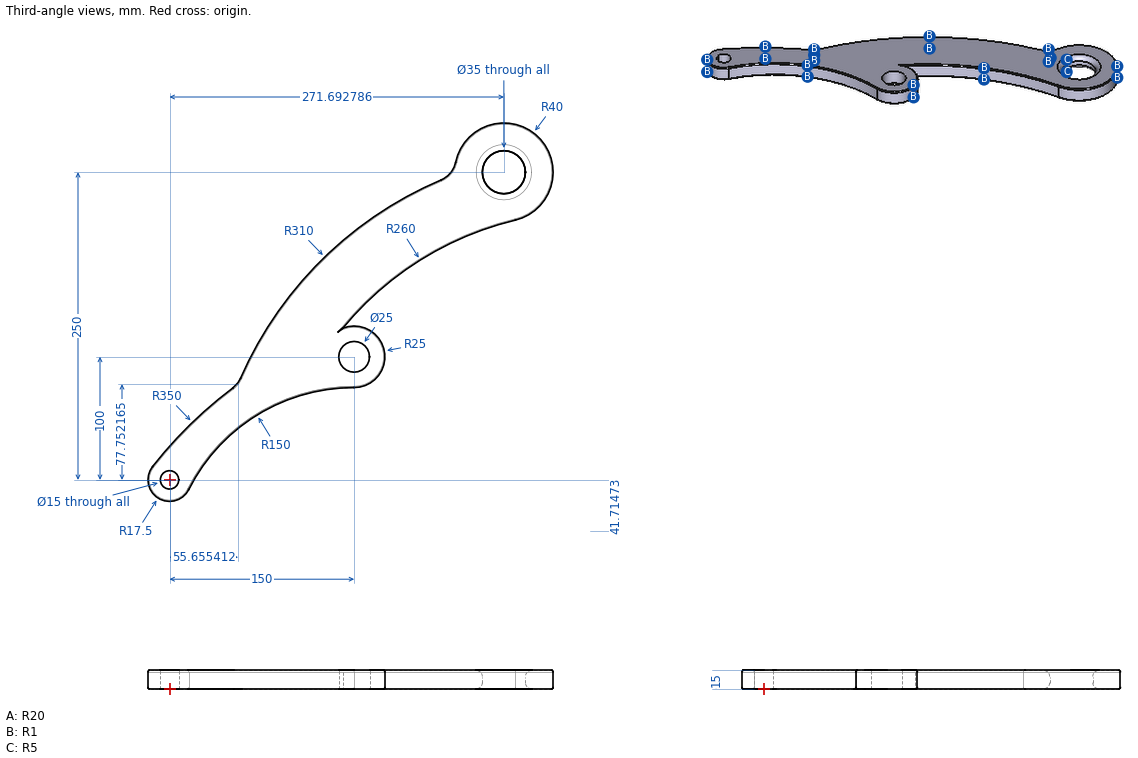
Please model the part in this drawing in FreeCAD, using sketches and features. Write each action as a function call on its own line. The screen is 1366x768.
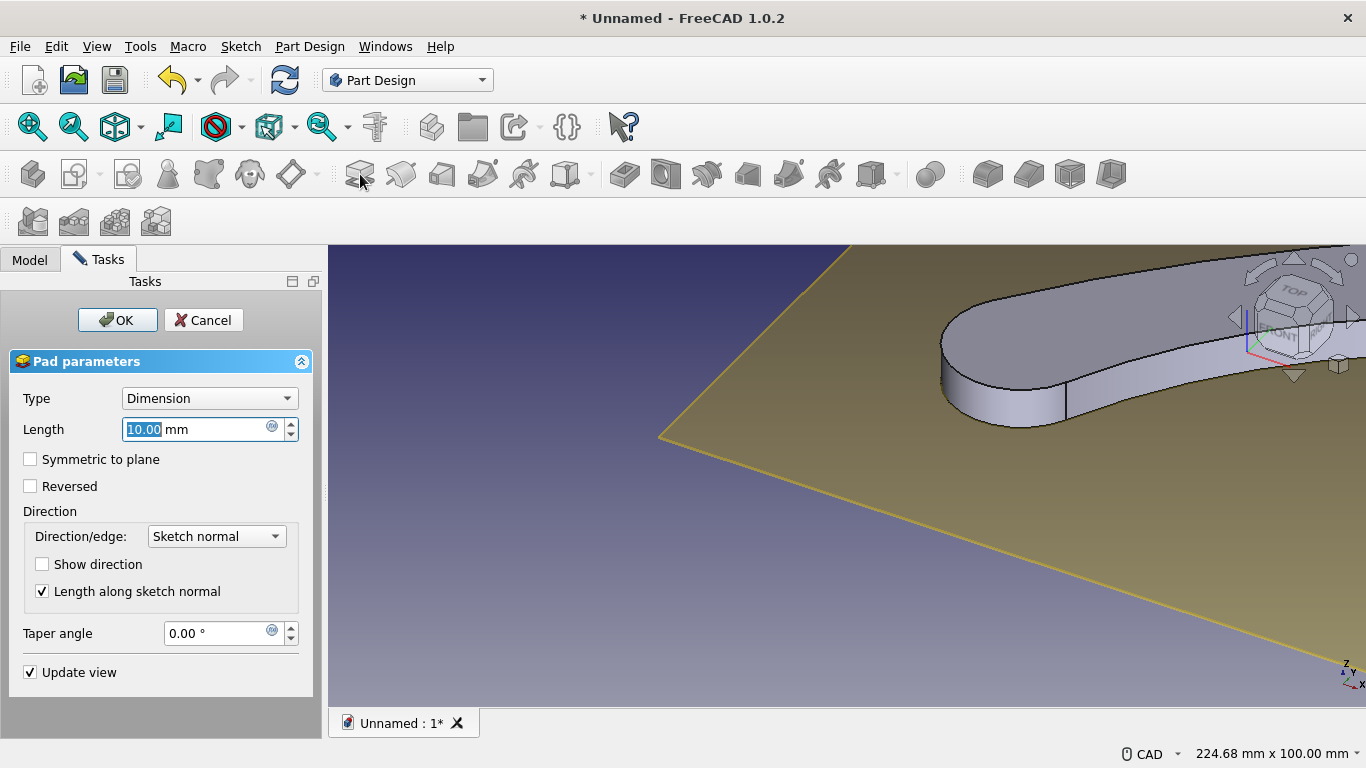
text(15)
key(Tab)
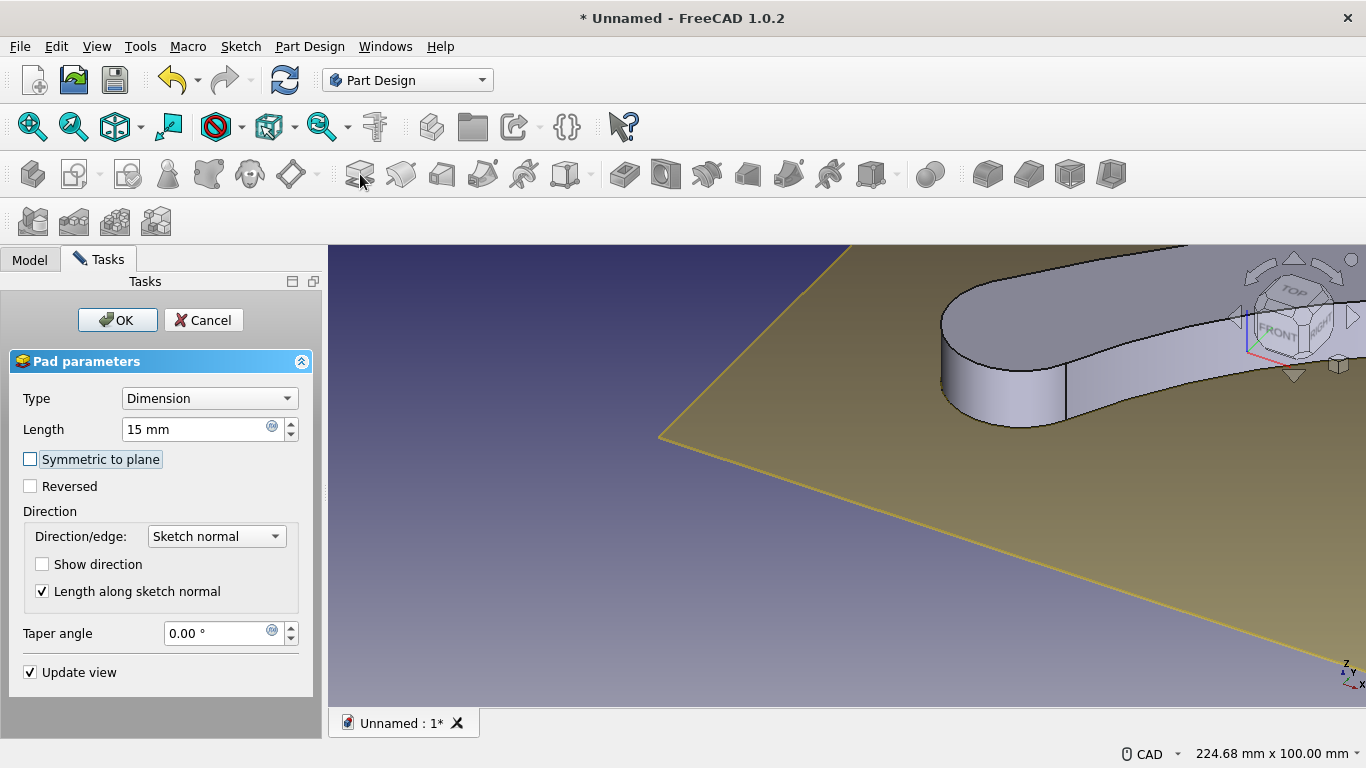
click(31, 486)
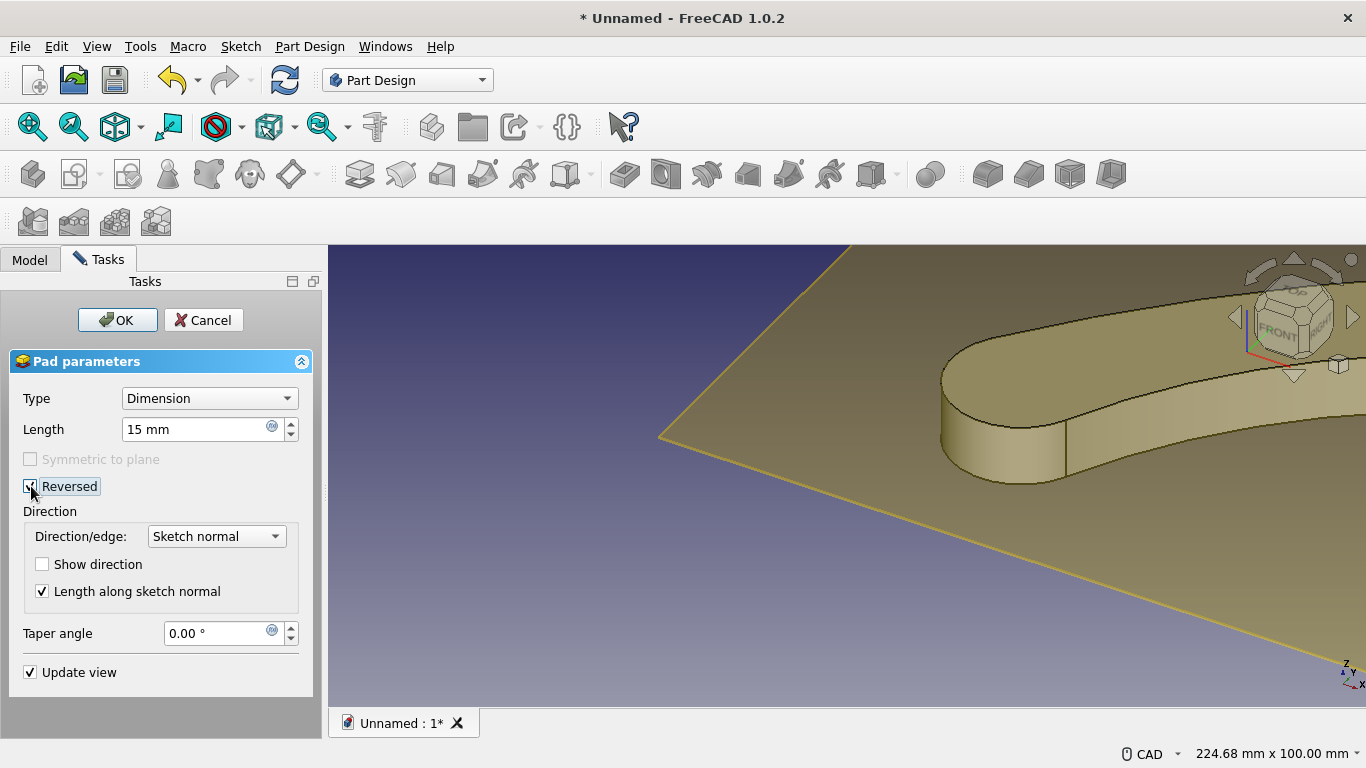
click(118, 320)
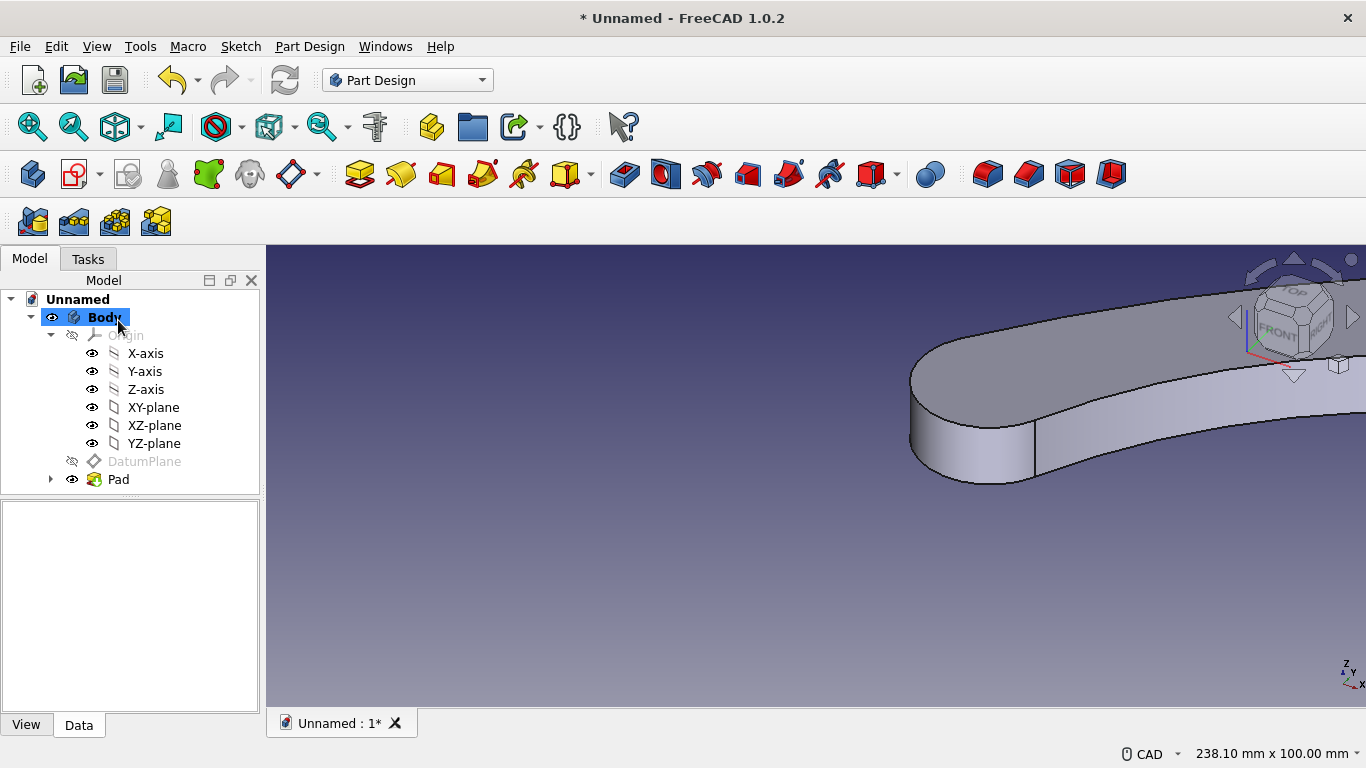
click(33, 128)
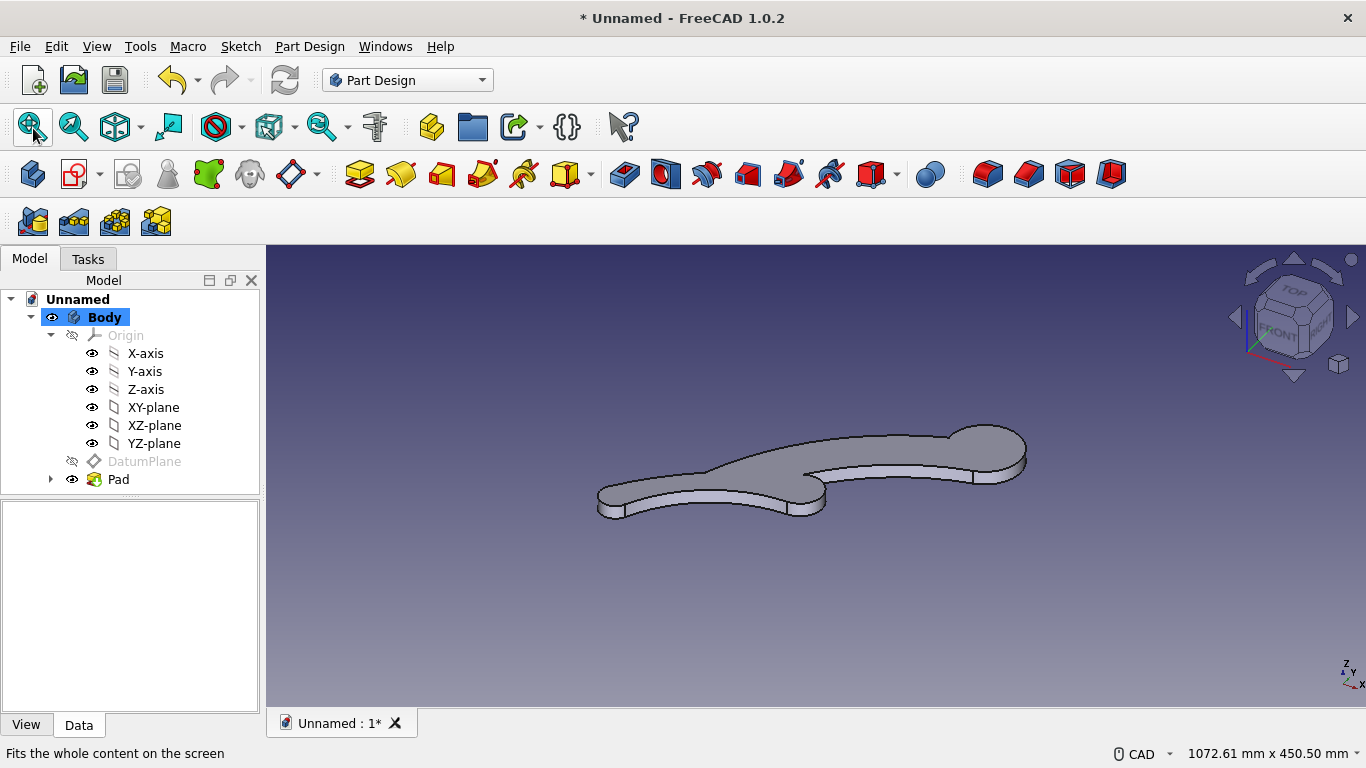
key(5)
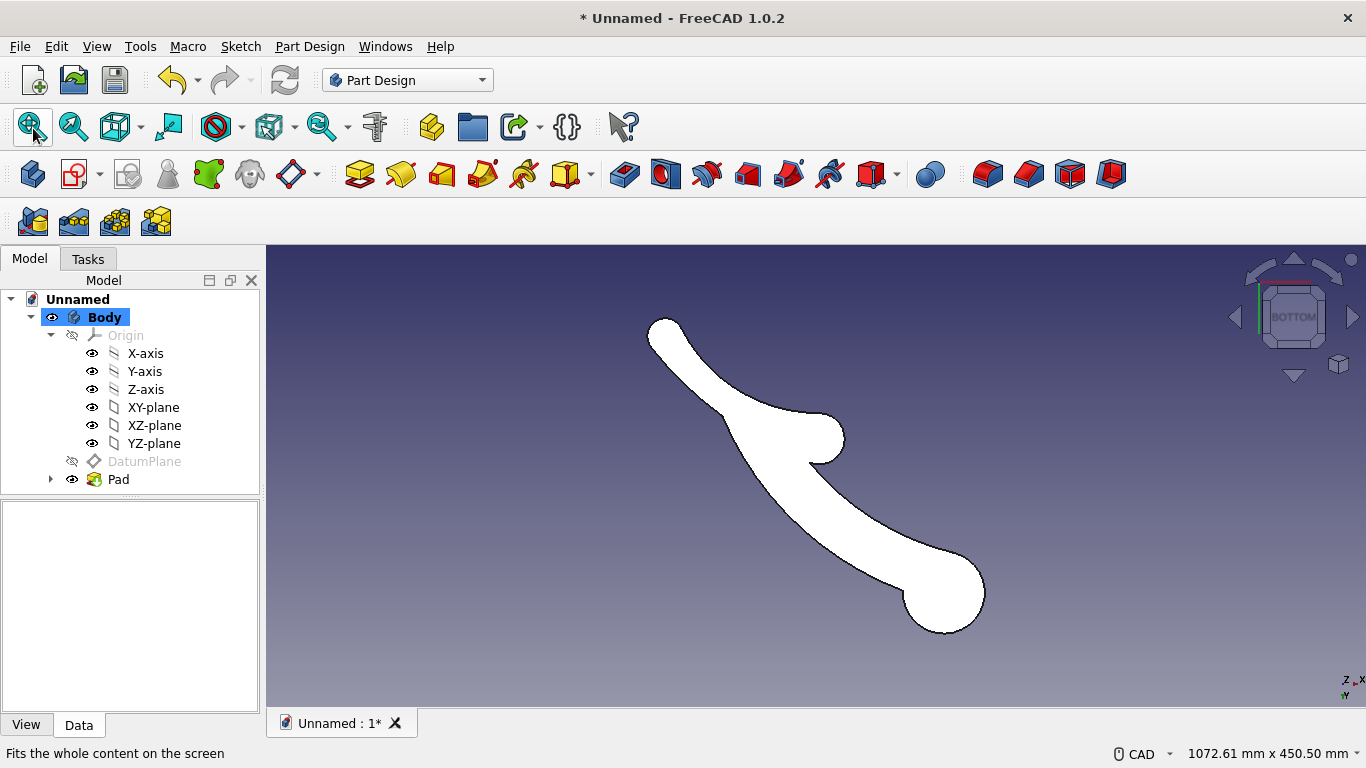
click(768, 430)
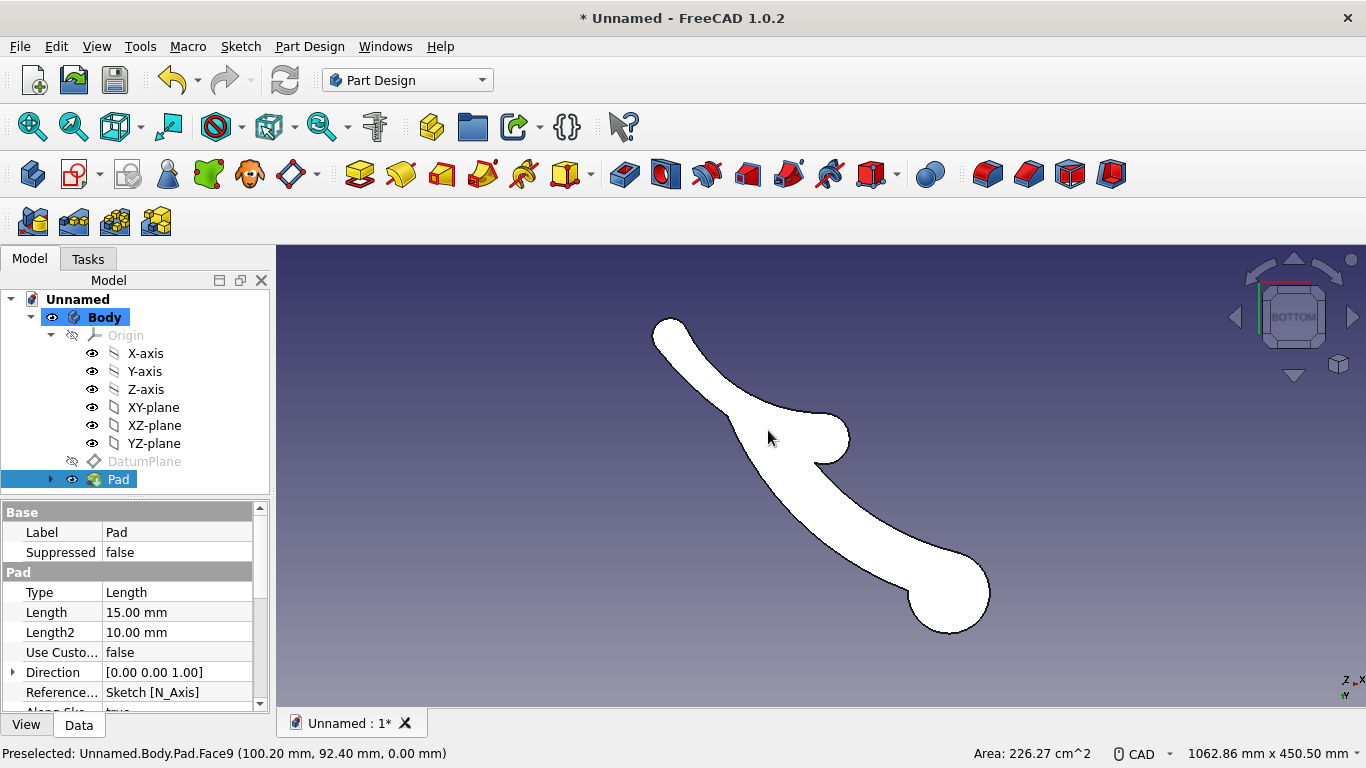
click(74, 174)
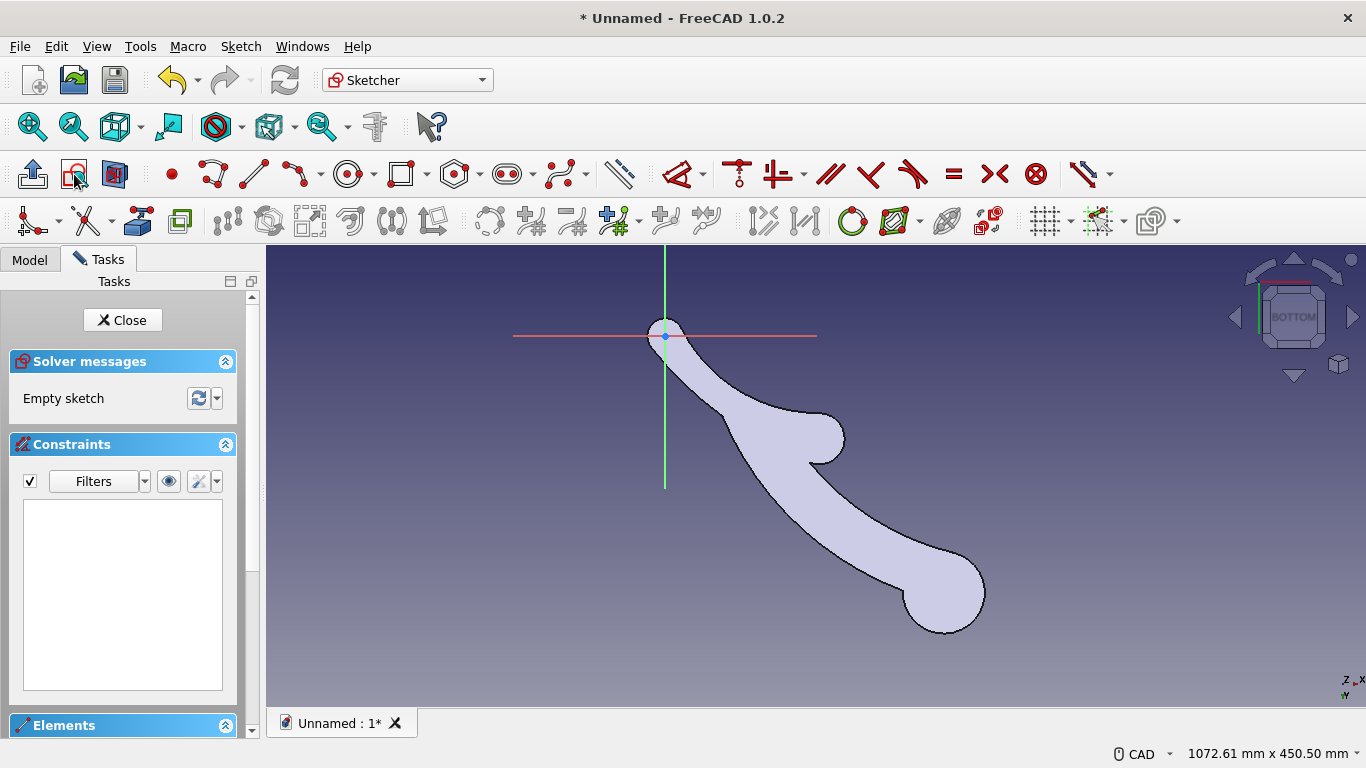
scroll(975, 611, up, 10)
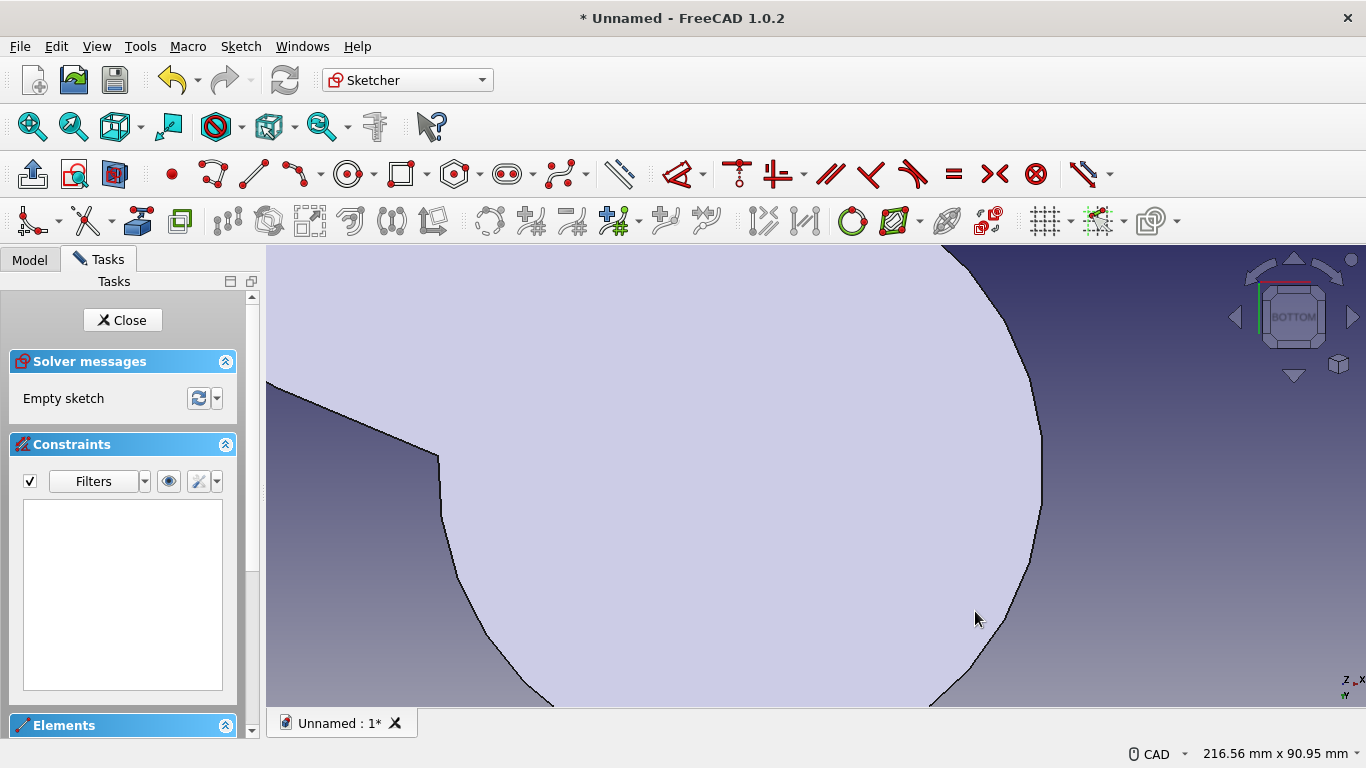
click(348, 174)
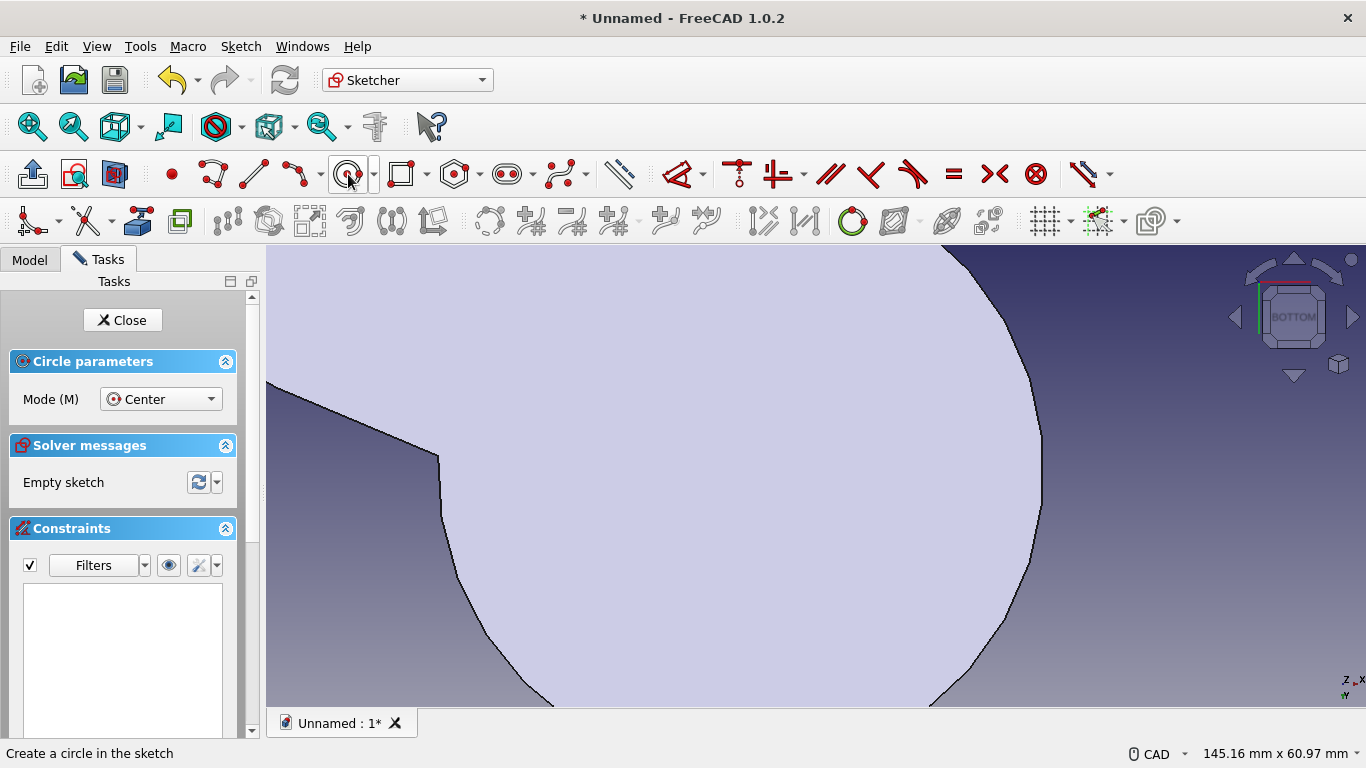
click(741, 470)
move(835, 376)